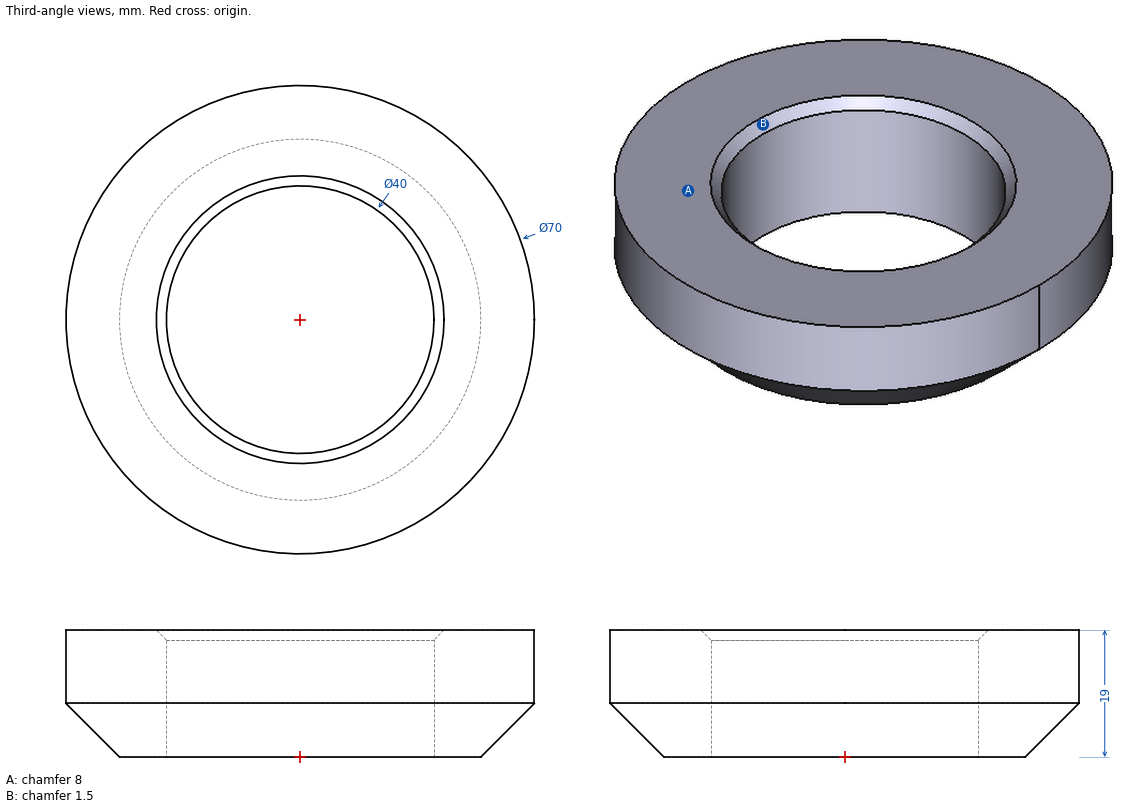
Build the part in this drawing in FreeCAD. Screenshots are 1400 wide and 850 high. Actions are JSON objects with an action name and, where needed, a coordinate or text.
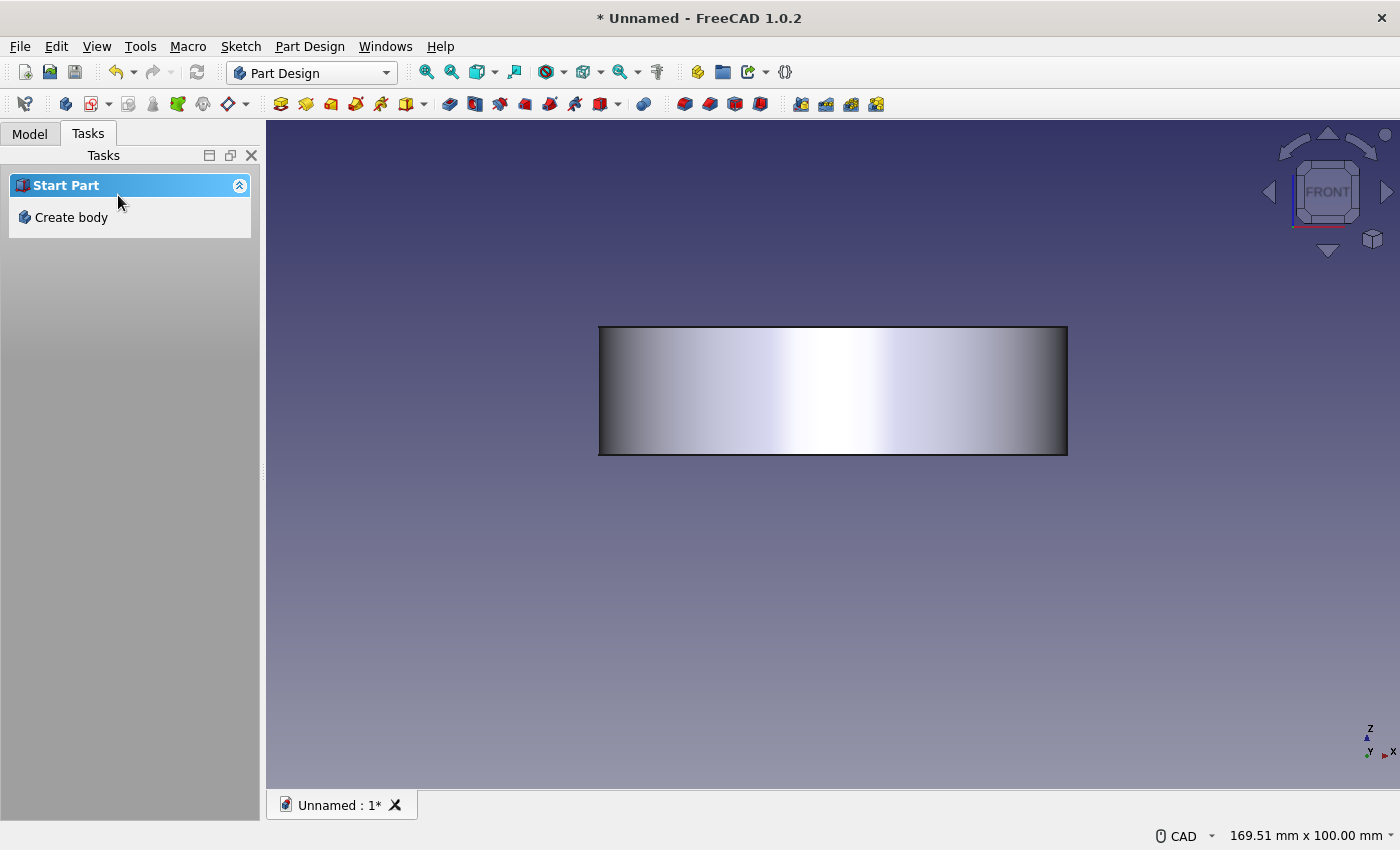
{"action": "left_click", "coordinate": [427, 72]}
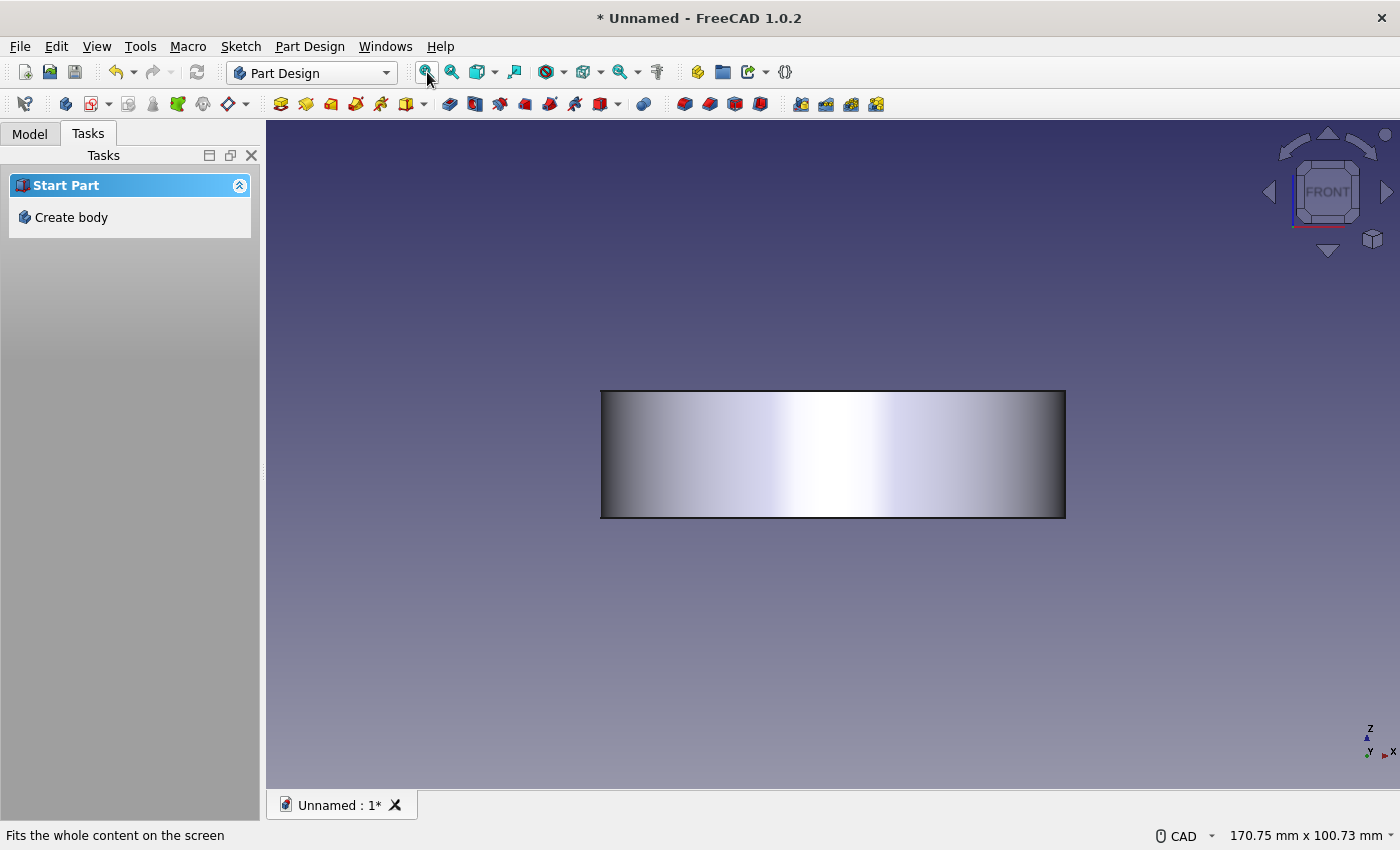
{"action": "left_click", "coordinate": [645, 517]}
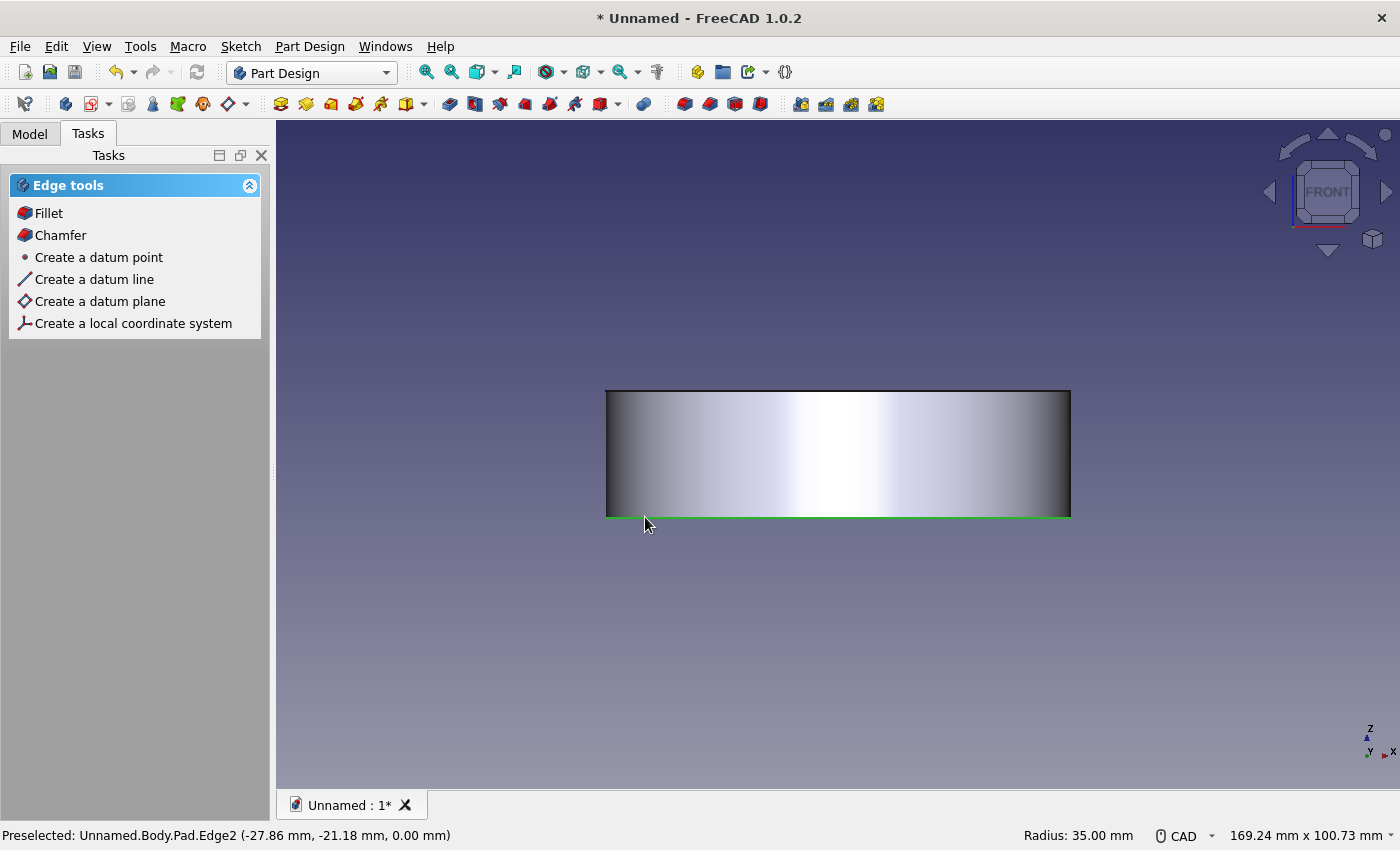
{"action": "left_click", "coordinate": [710, 104]}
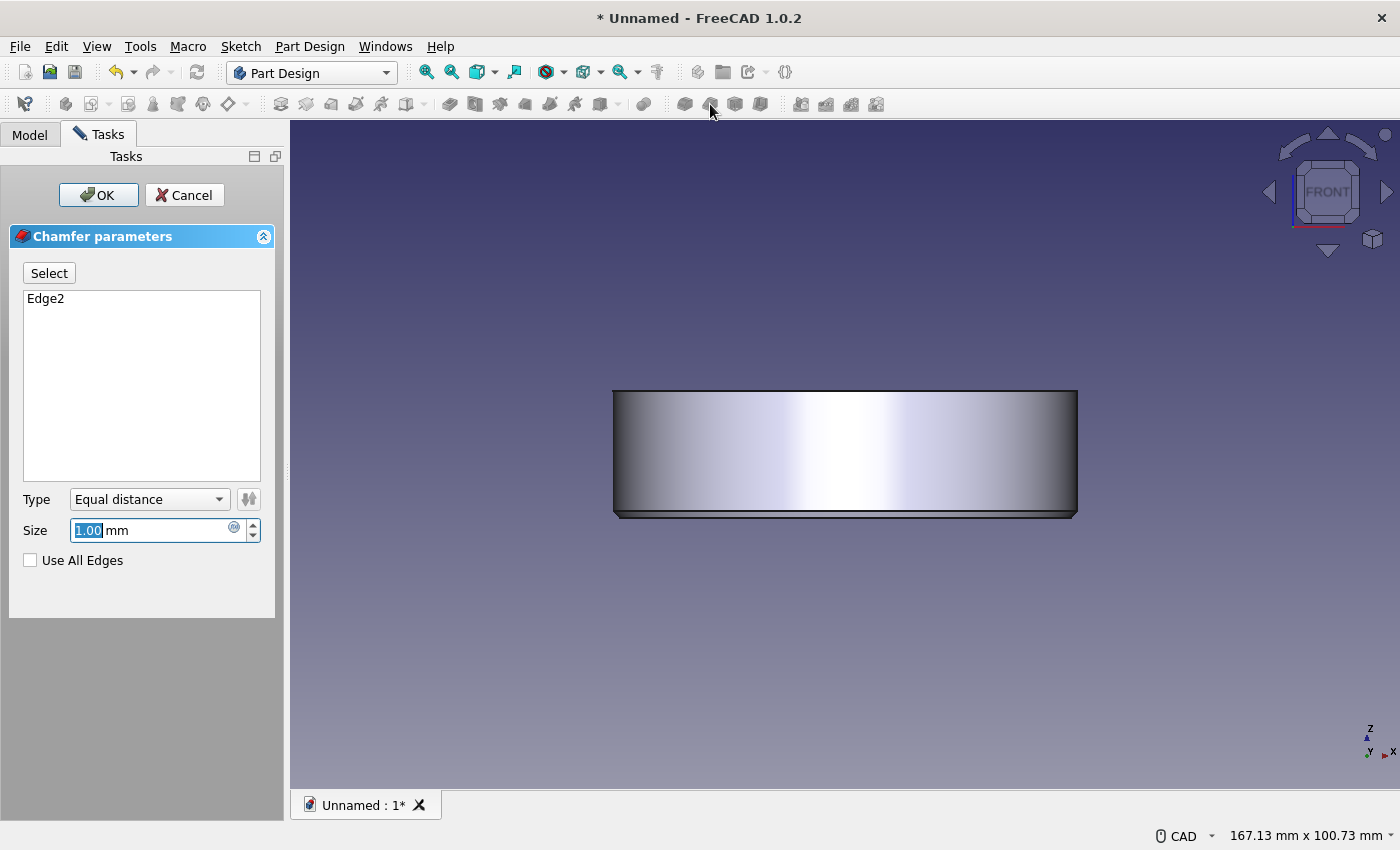
{"action": "type", "text": "8"}
{"action": "key", "text": "Tab"}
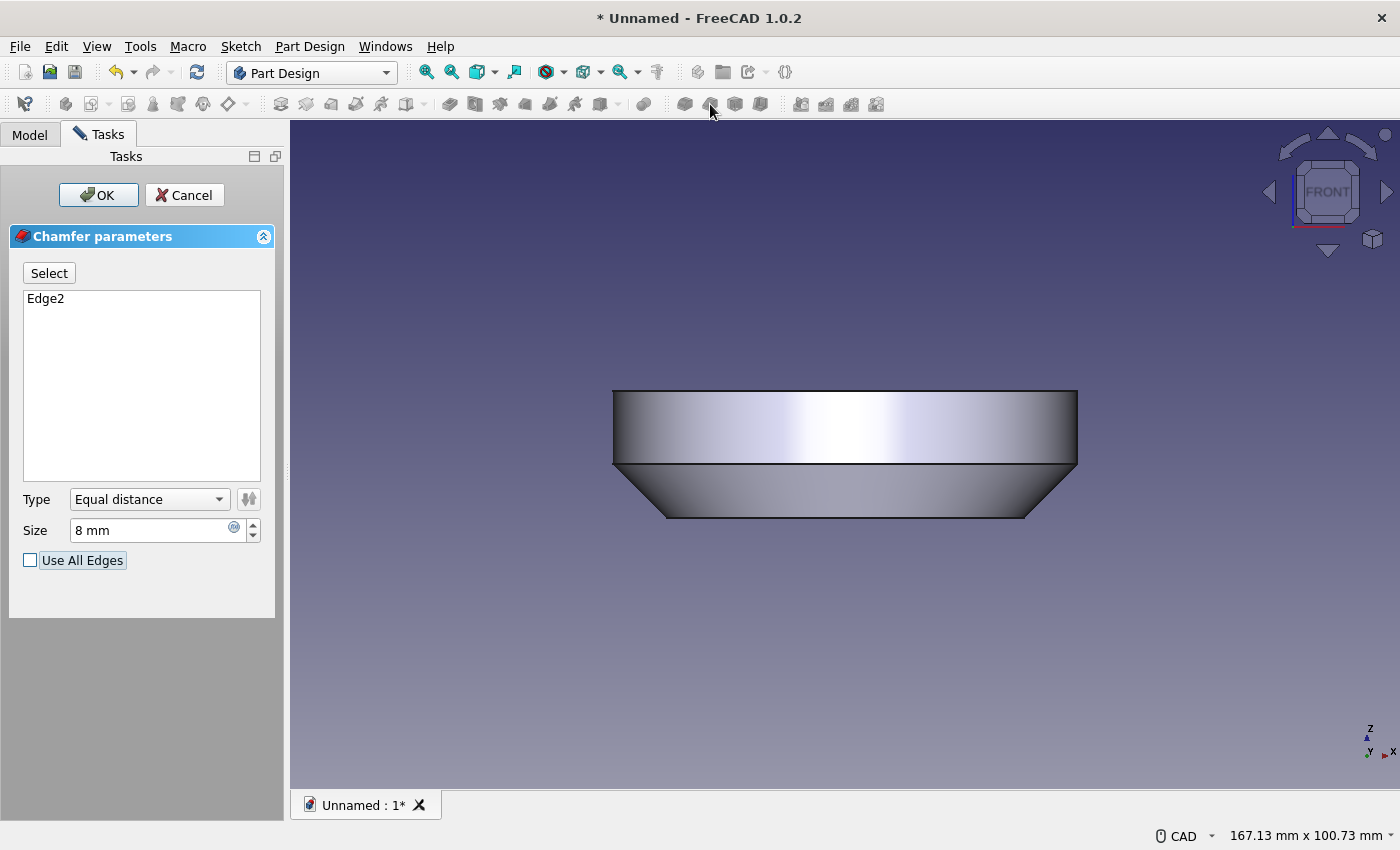
{"action": "left_click", "coordinate": [99, 195]}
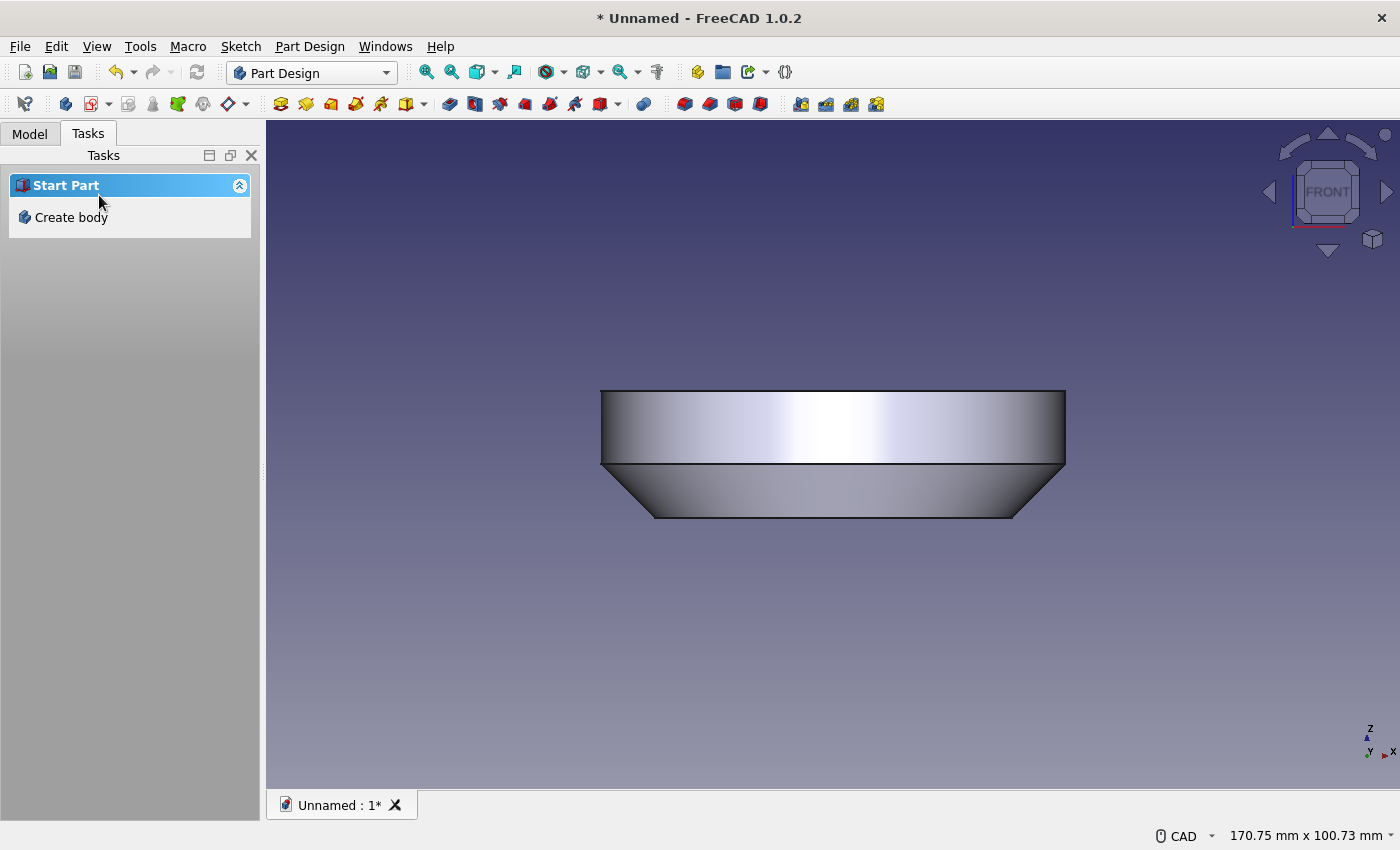
{"action": "key", "text": "v f"}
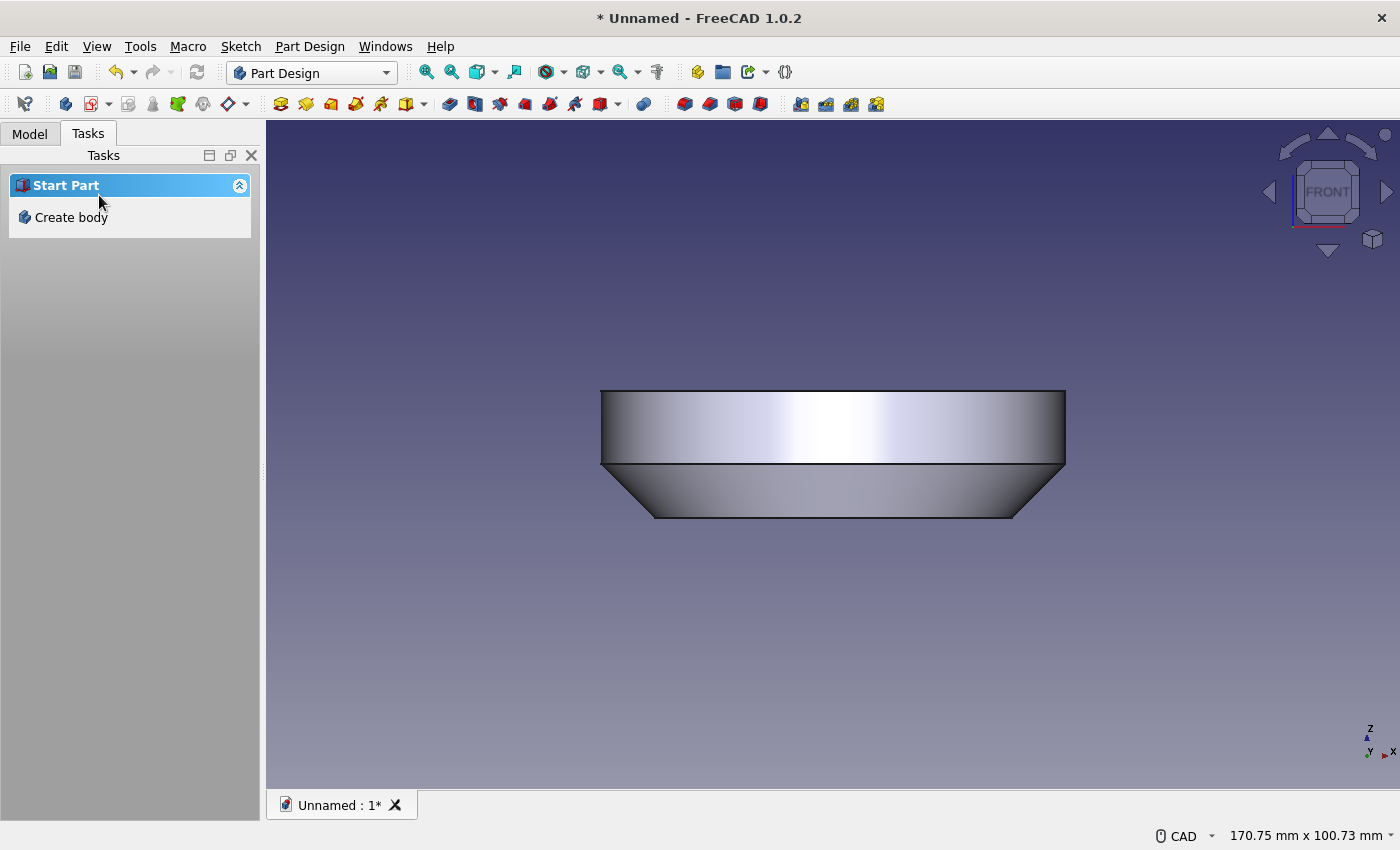
{"action": "key", "text": "0"}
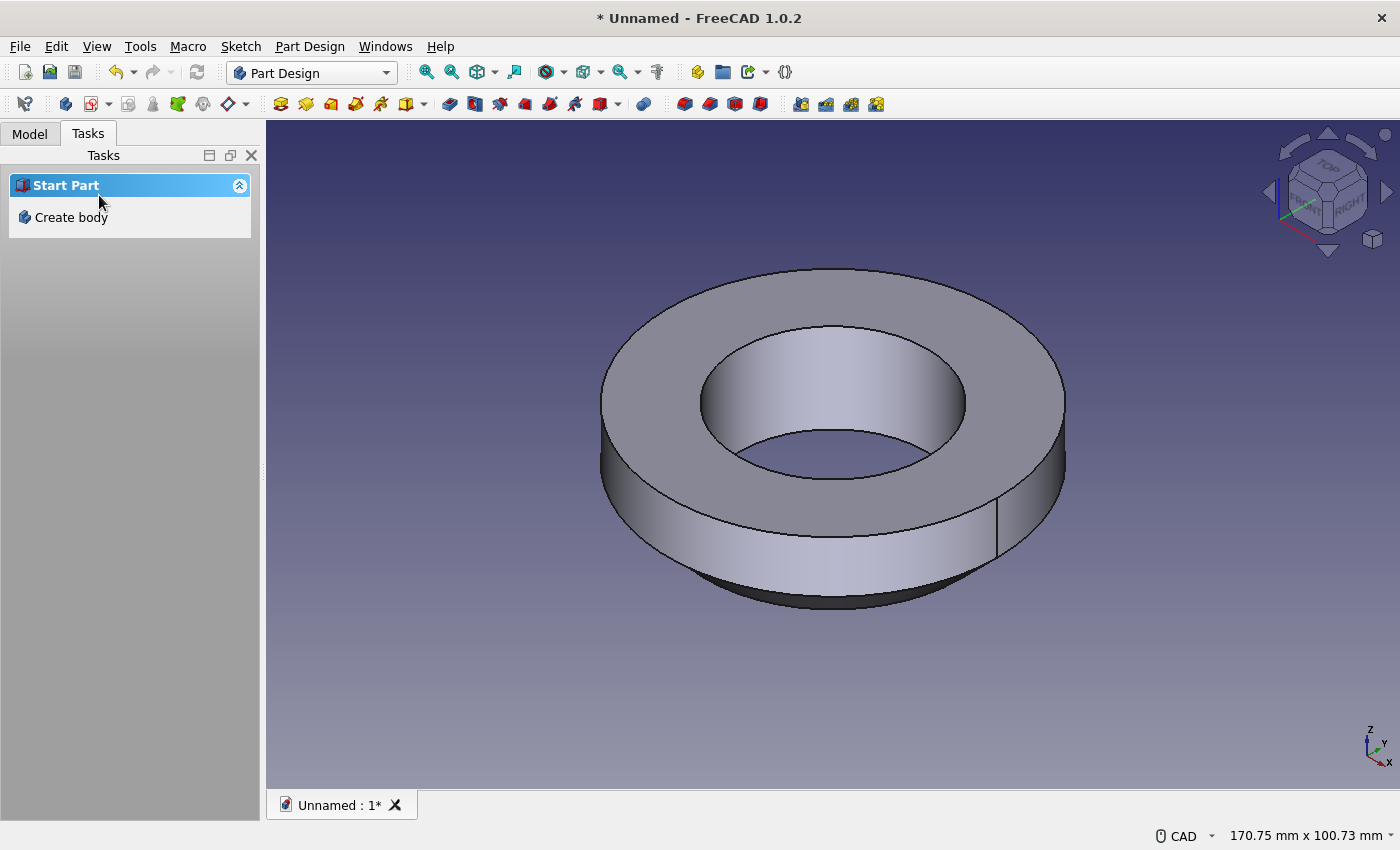
{"action": "left_click", "coordinate": [739, 348]}